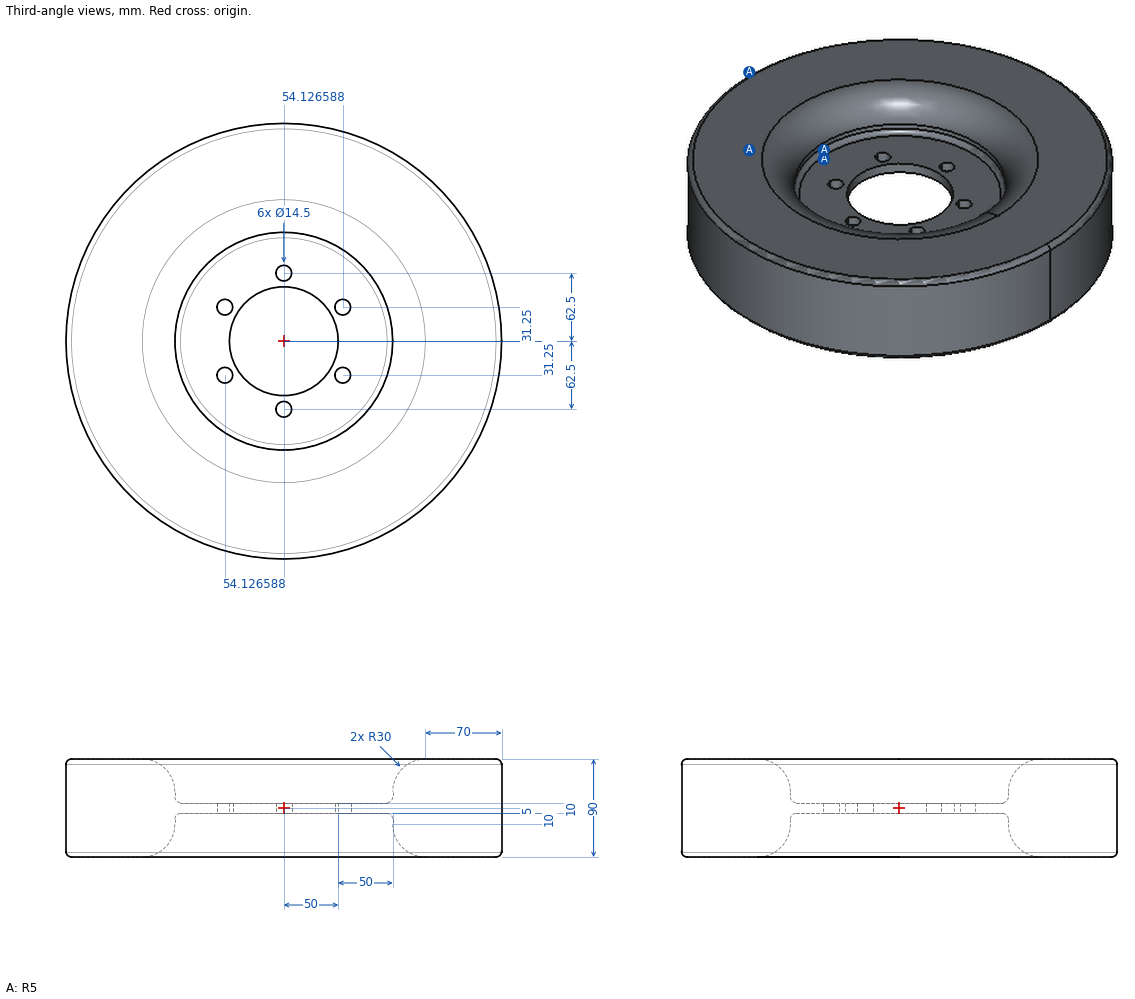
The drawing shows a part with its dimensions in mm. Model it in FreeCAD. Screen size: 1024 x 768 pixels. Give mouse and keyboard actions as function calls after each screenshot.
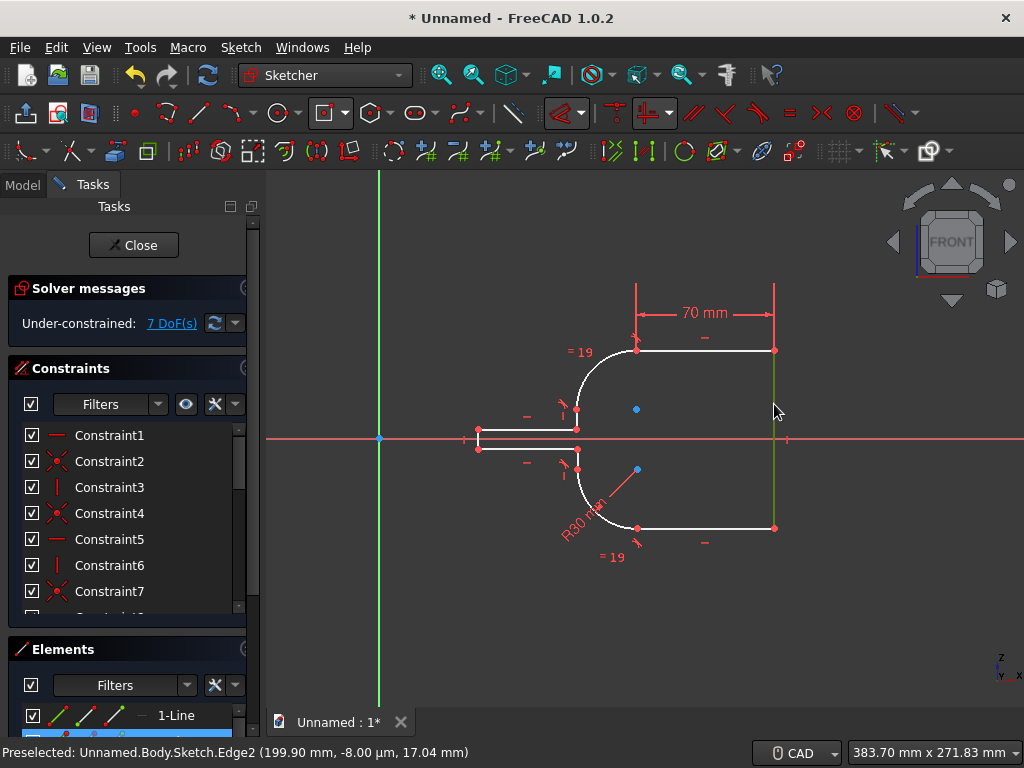
click(584, 114)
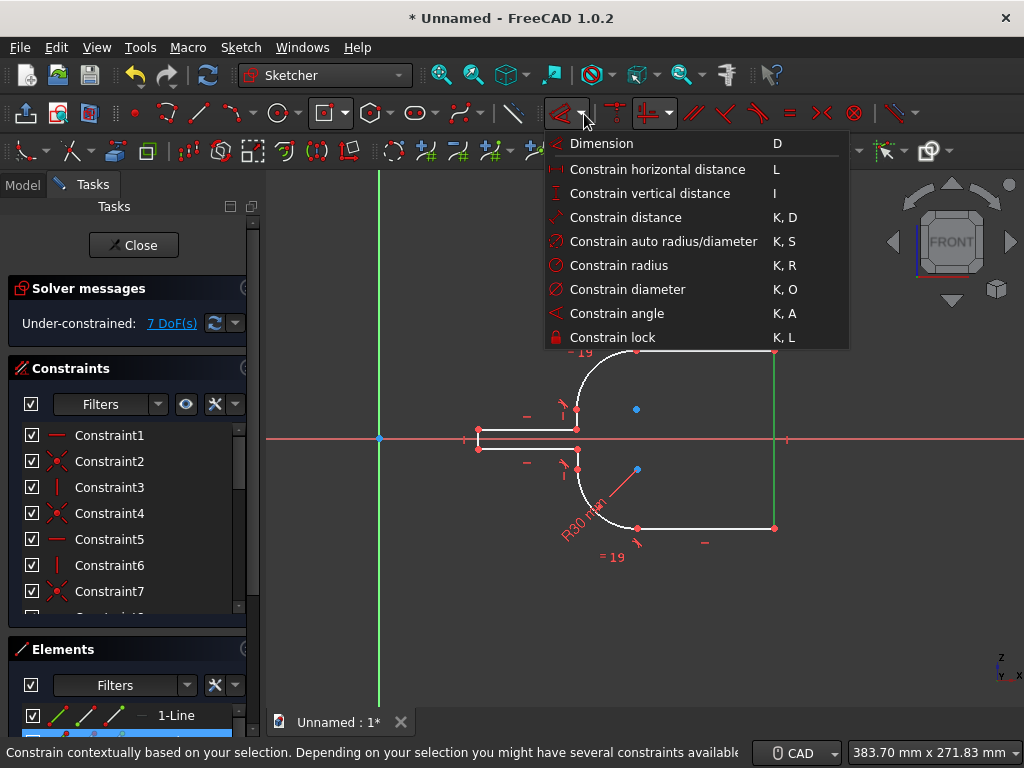
click(697, 193)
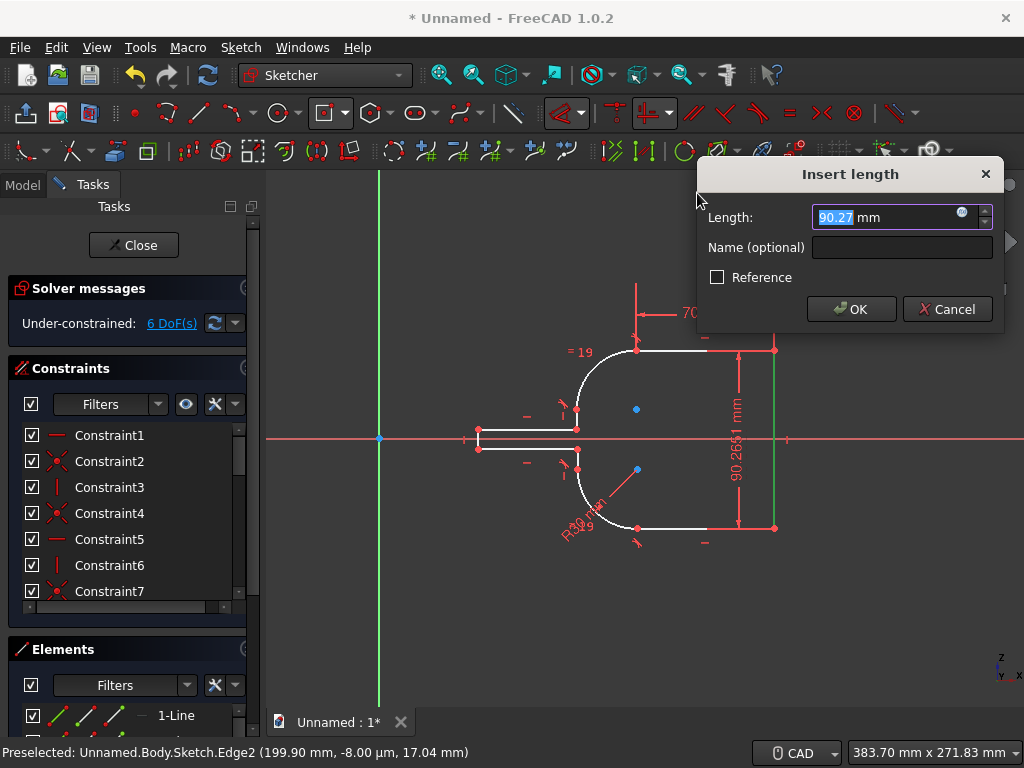
text(90)
key(Return)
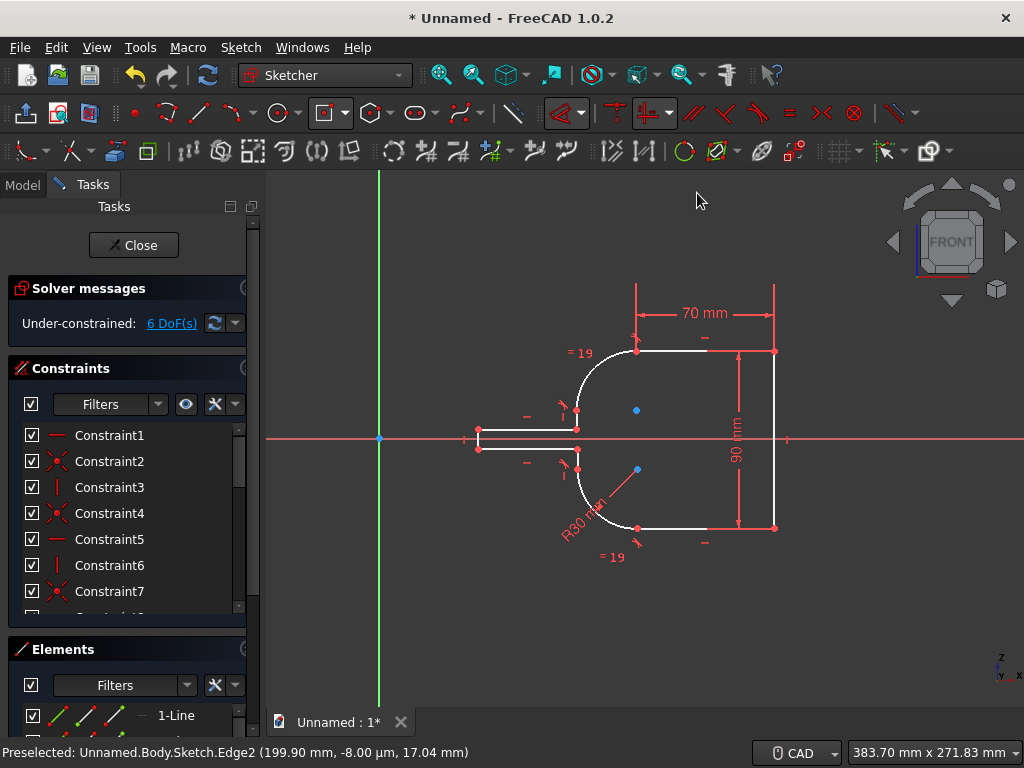
click(733, 529)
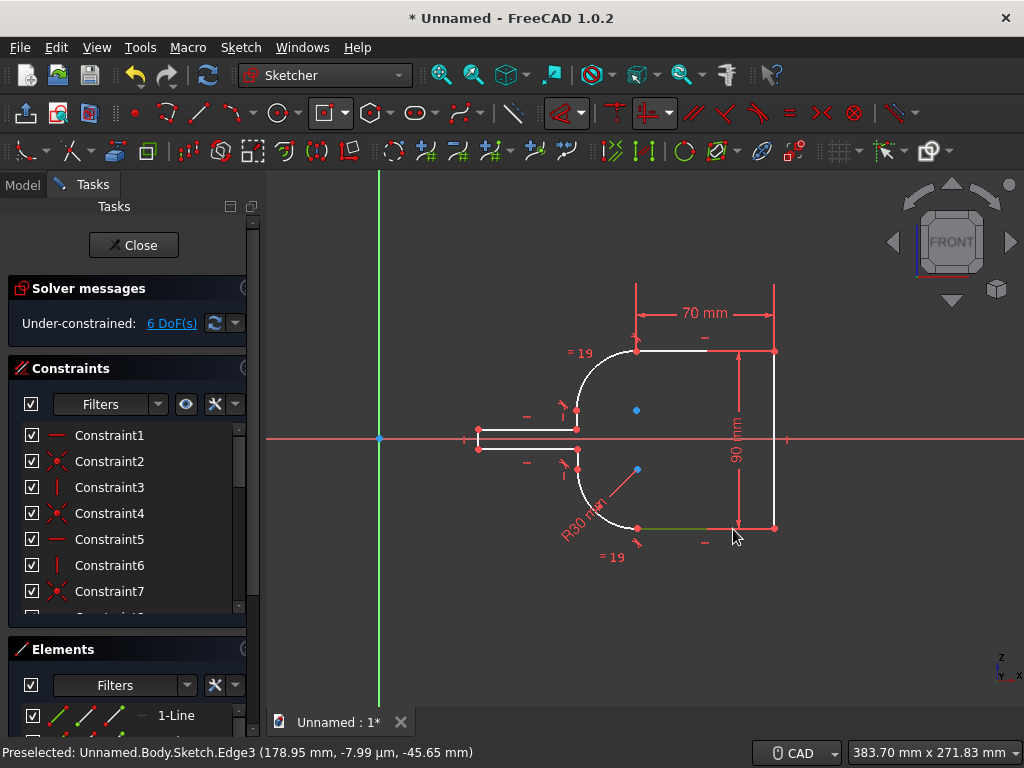
click(584, 114)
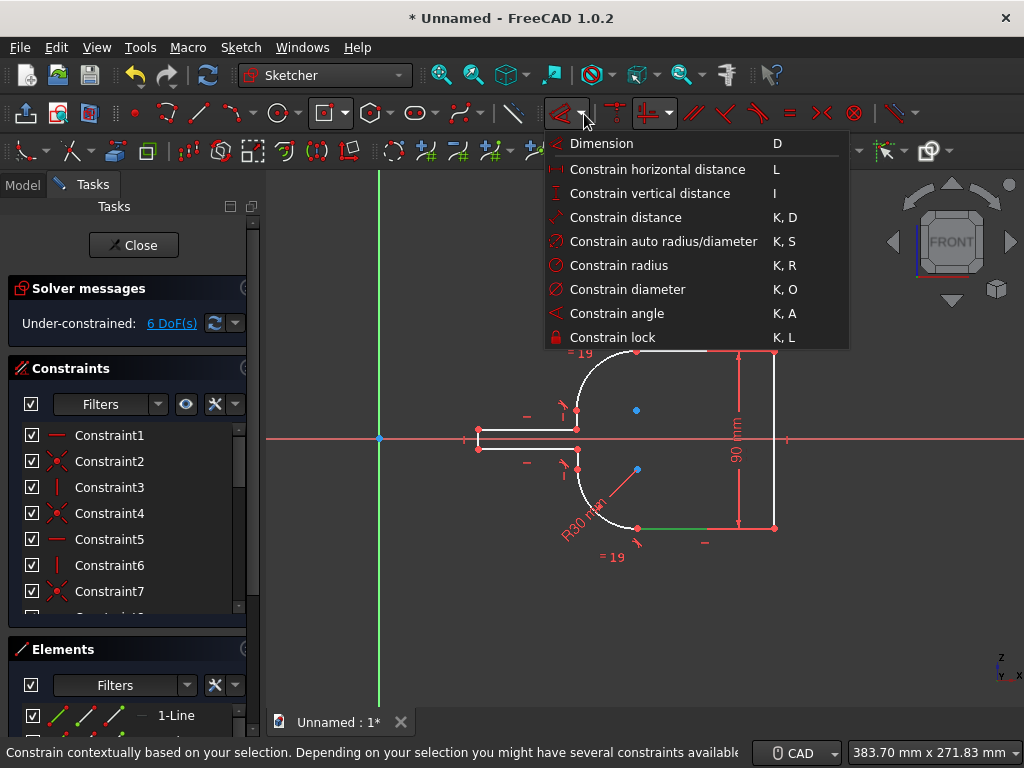
click(697, 169)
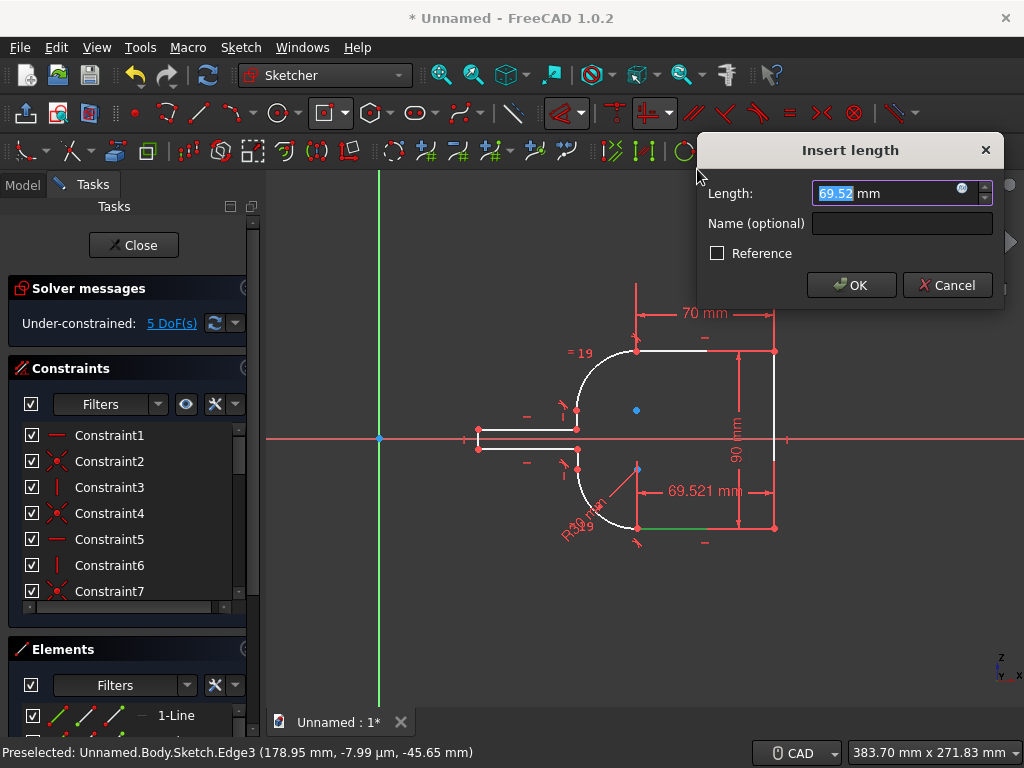
text(70)
key(Return)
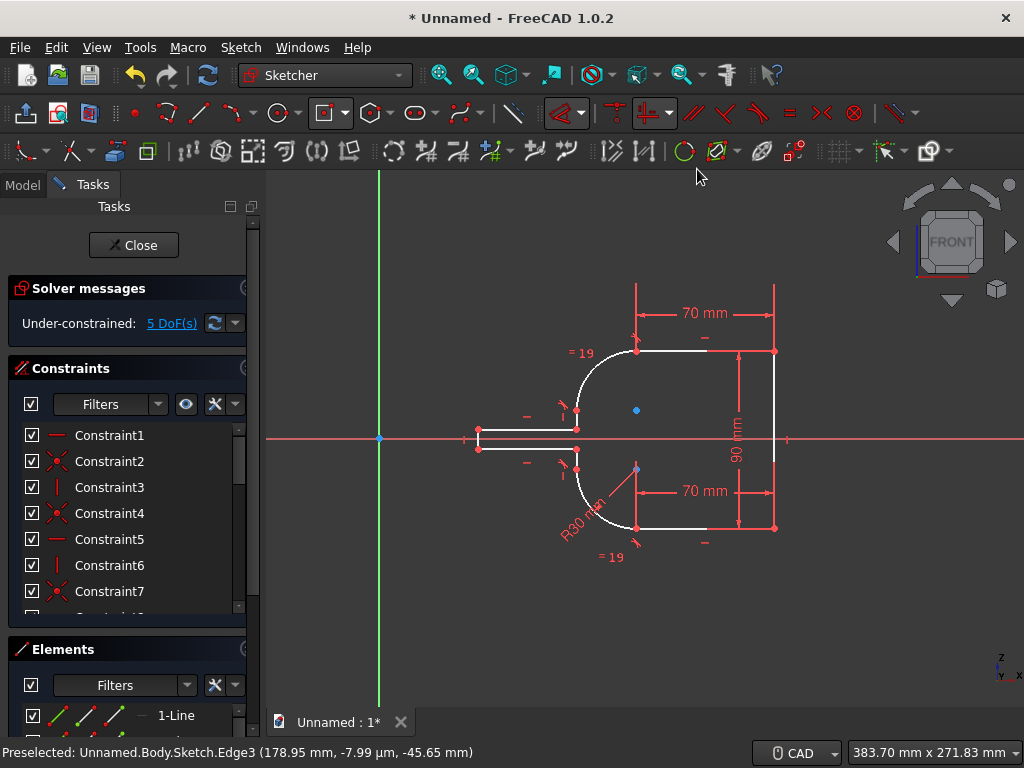
scroll(577, 459, up, 4)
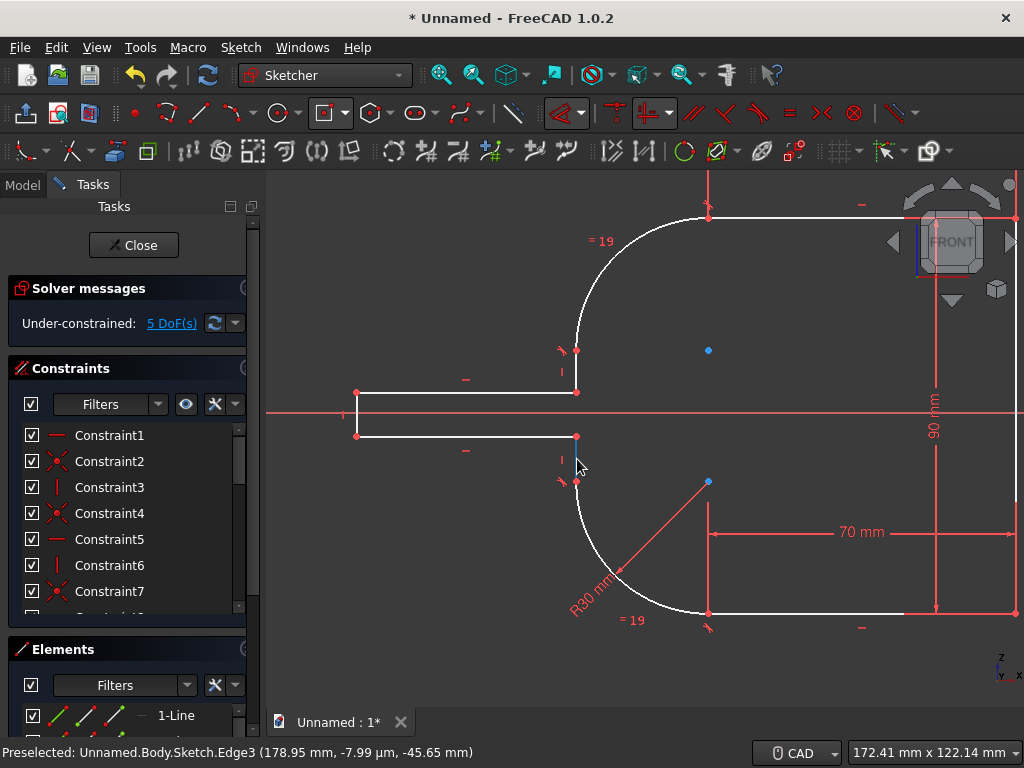
click(576, 459)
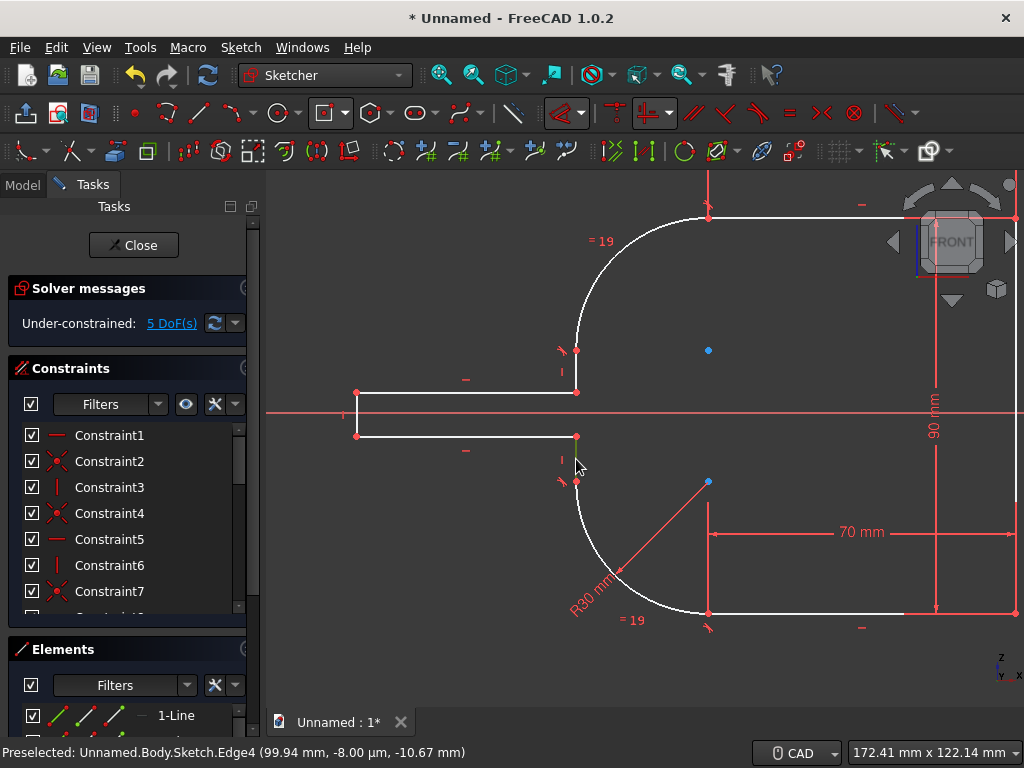
key(i)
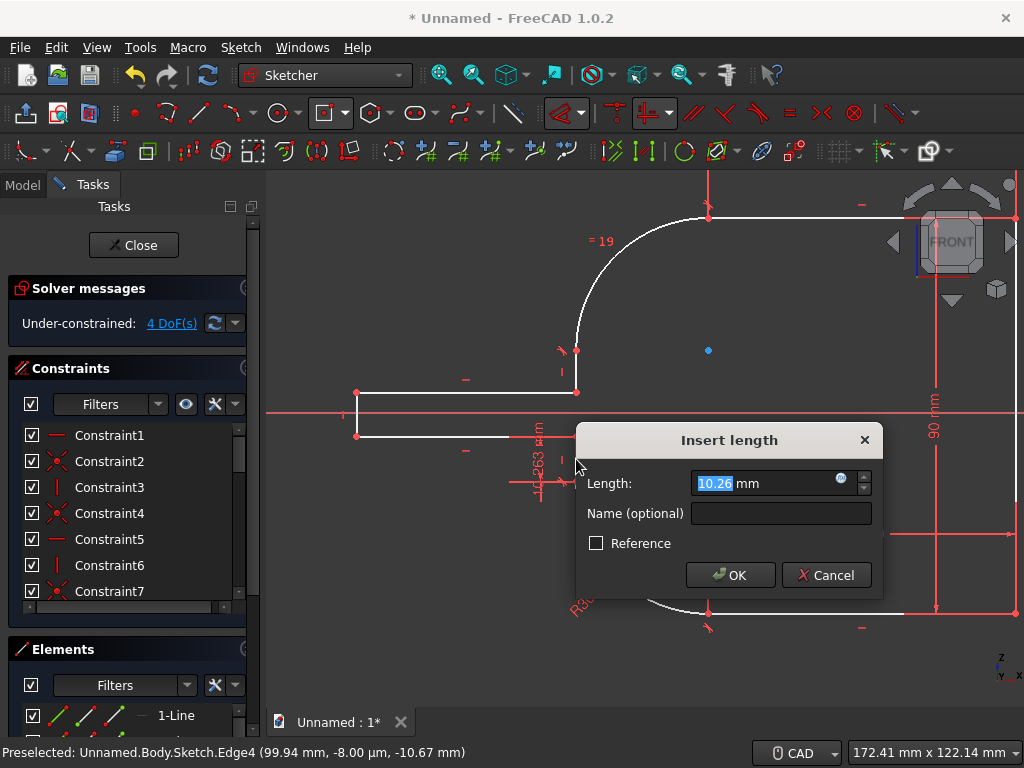
text(10)
key(Return)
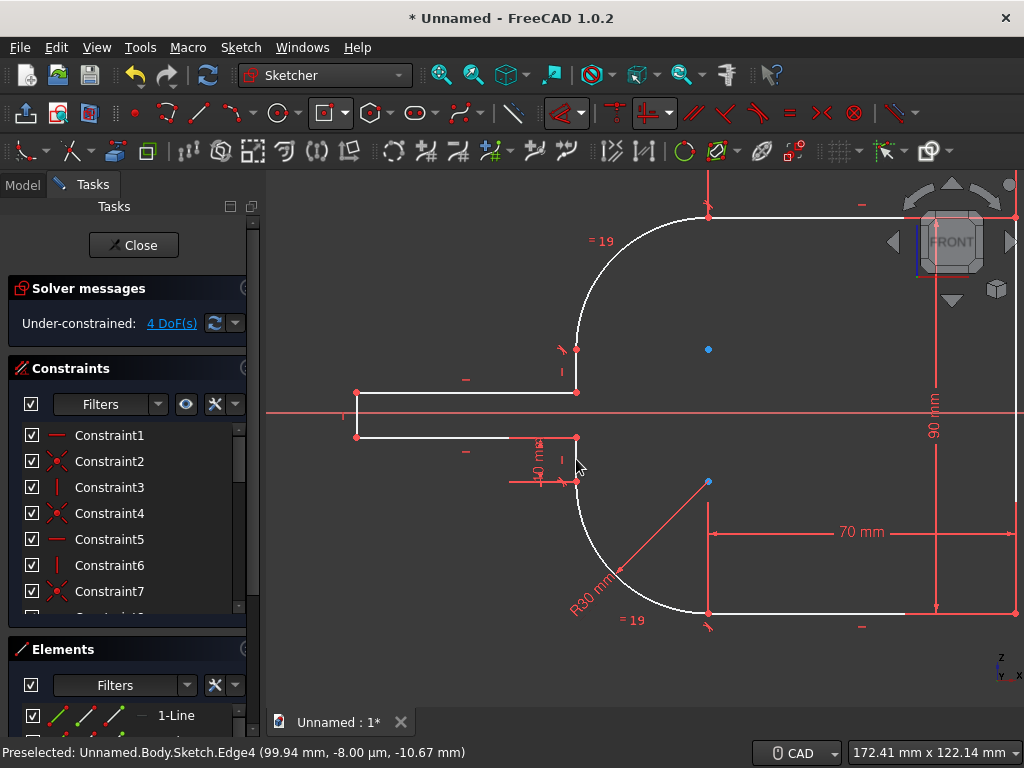
click(510, 438)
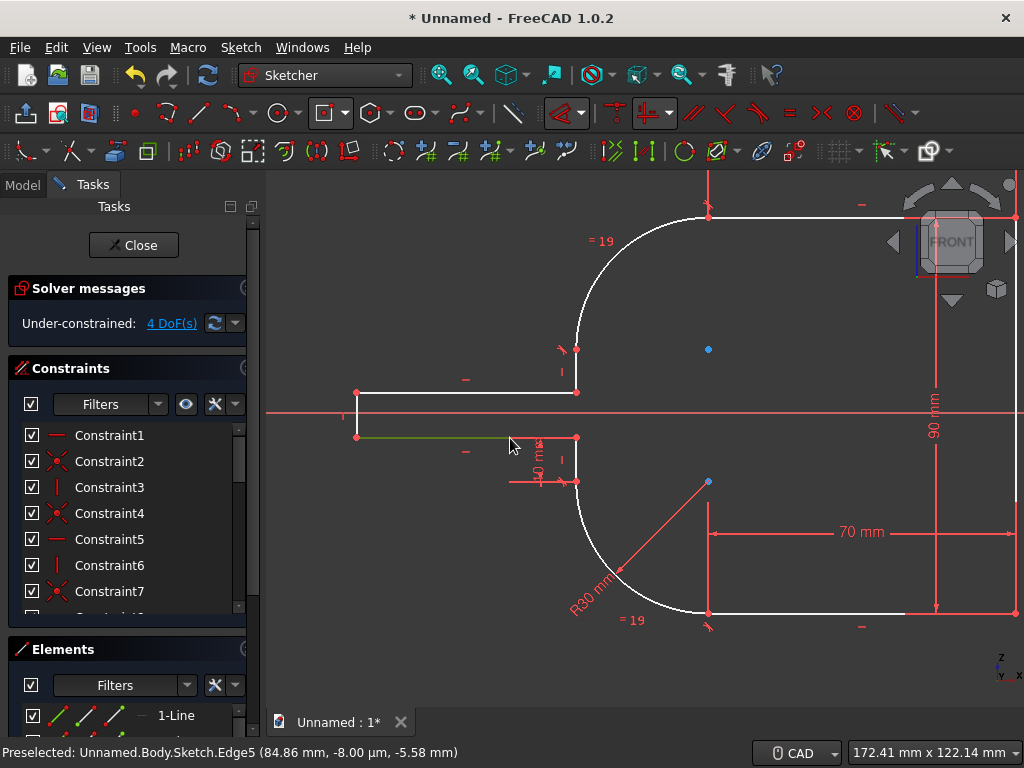
click(584, 114)